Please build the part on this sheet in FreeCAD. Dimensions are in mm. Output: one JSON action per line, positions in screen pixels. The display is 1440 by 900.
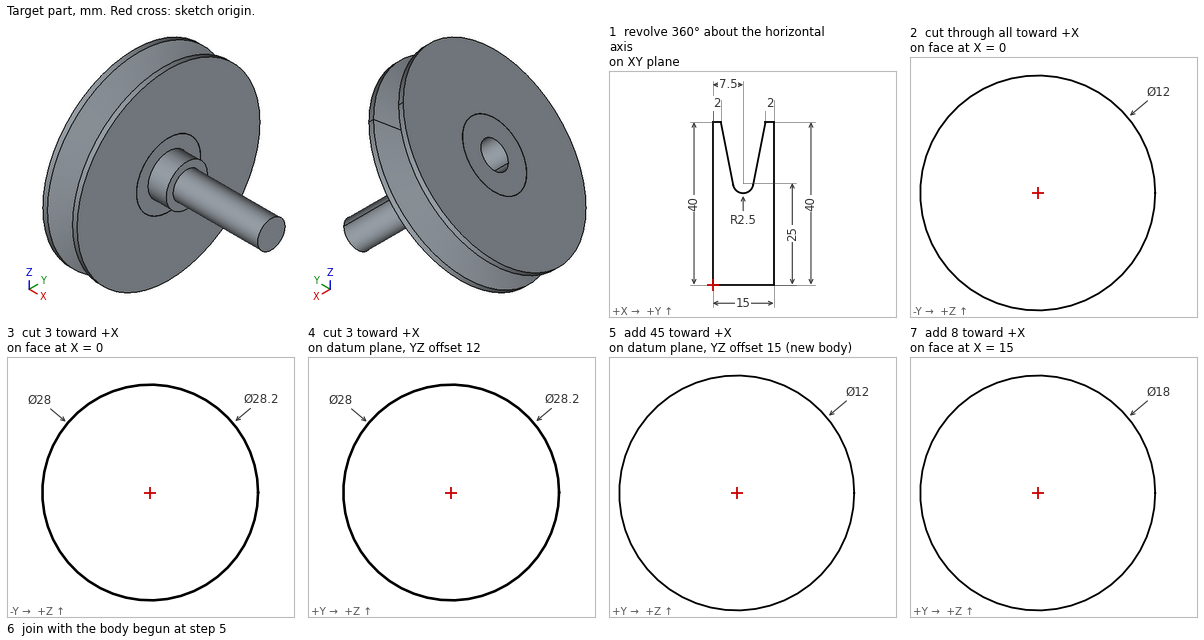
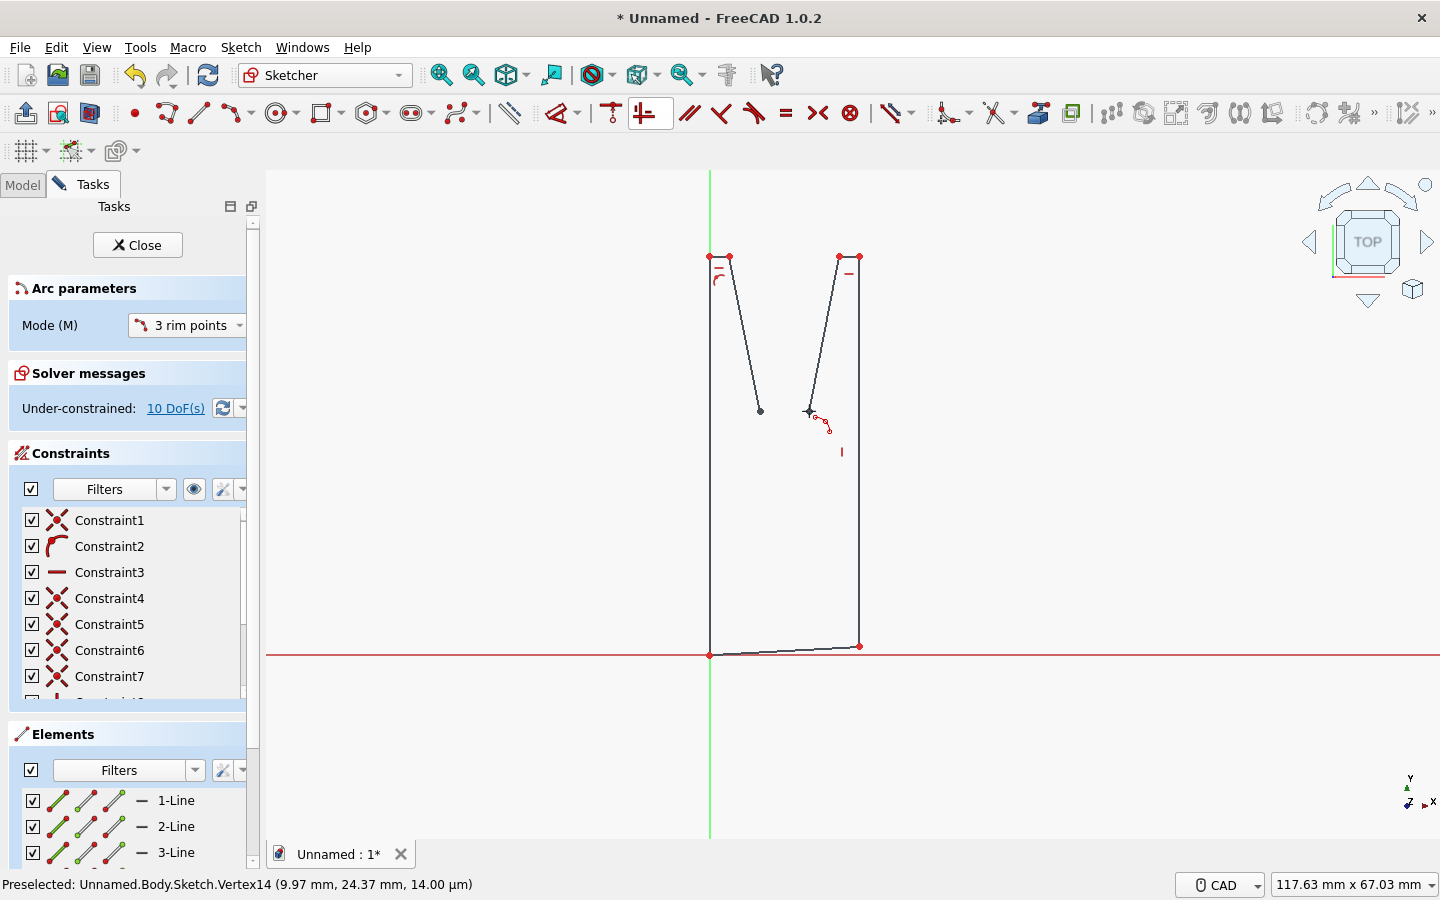
{"action": "left_click", "coordinate": [809, 412]}
{"action": "left_click", "coordinate": [760, 412]}
{"action": "left_click", "coordinate": [784, 431]}
{"action": "key", "text": "Escape"}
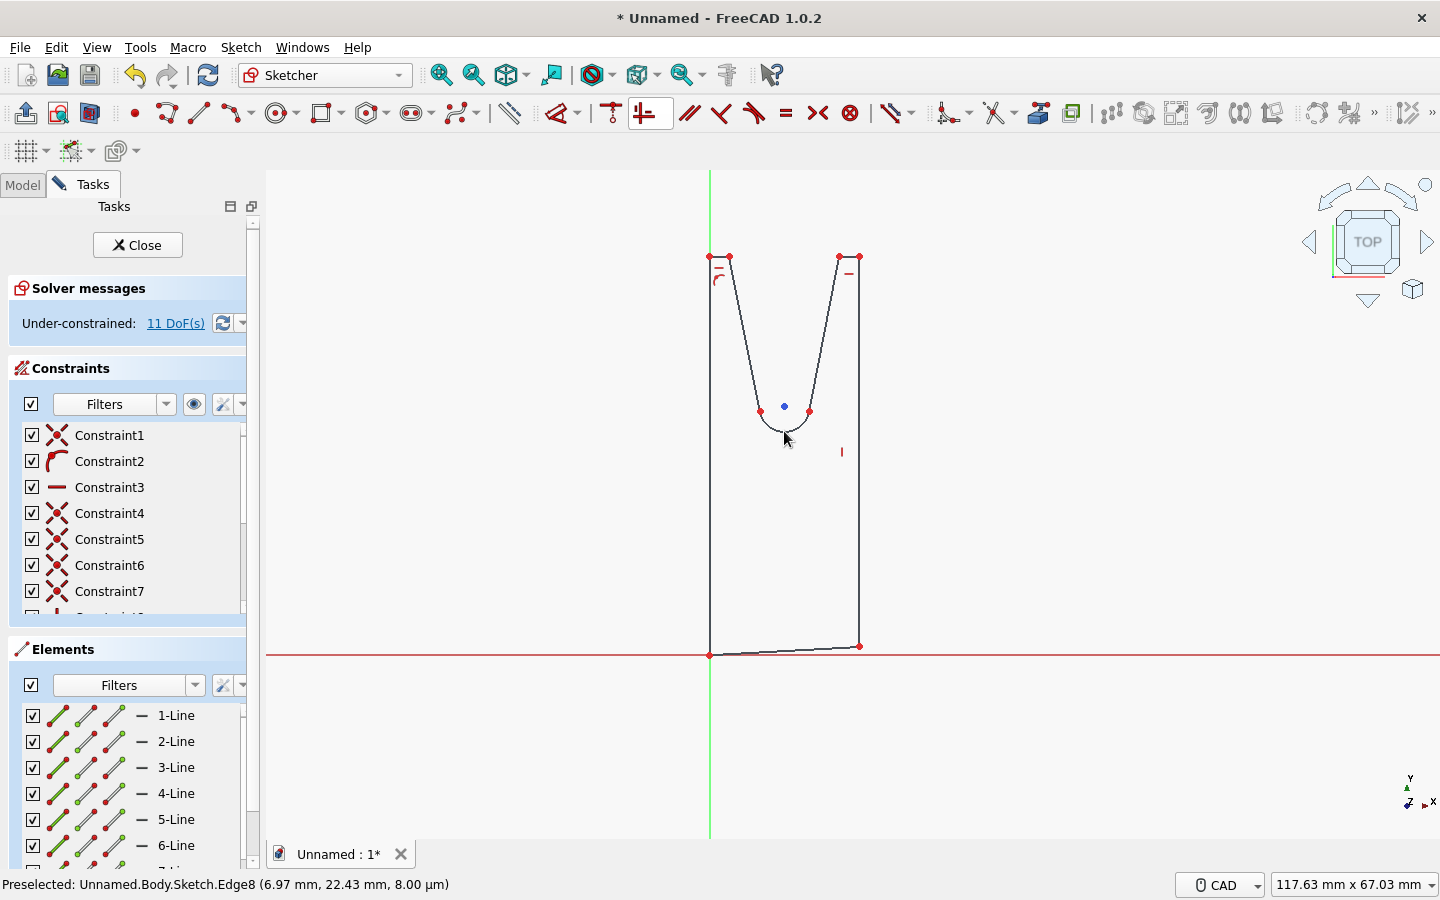
{"action": "left_click", "coordinate": [751, 365]}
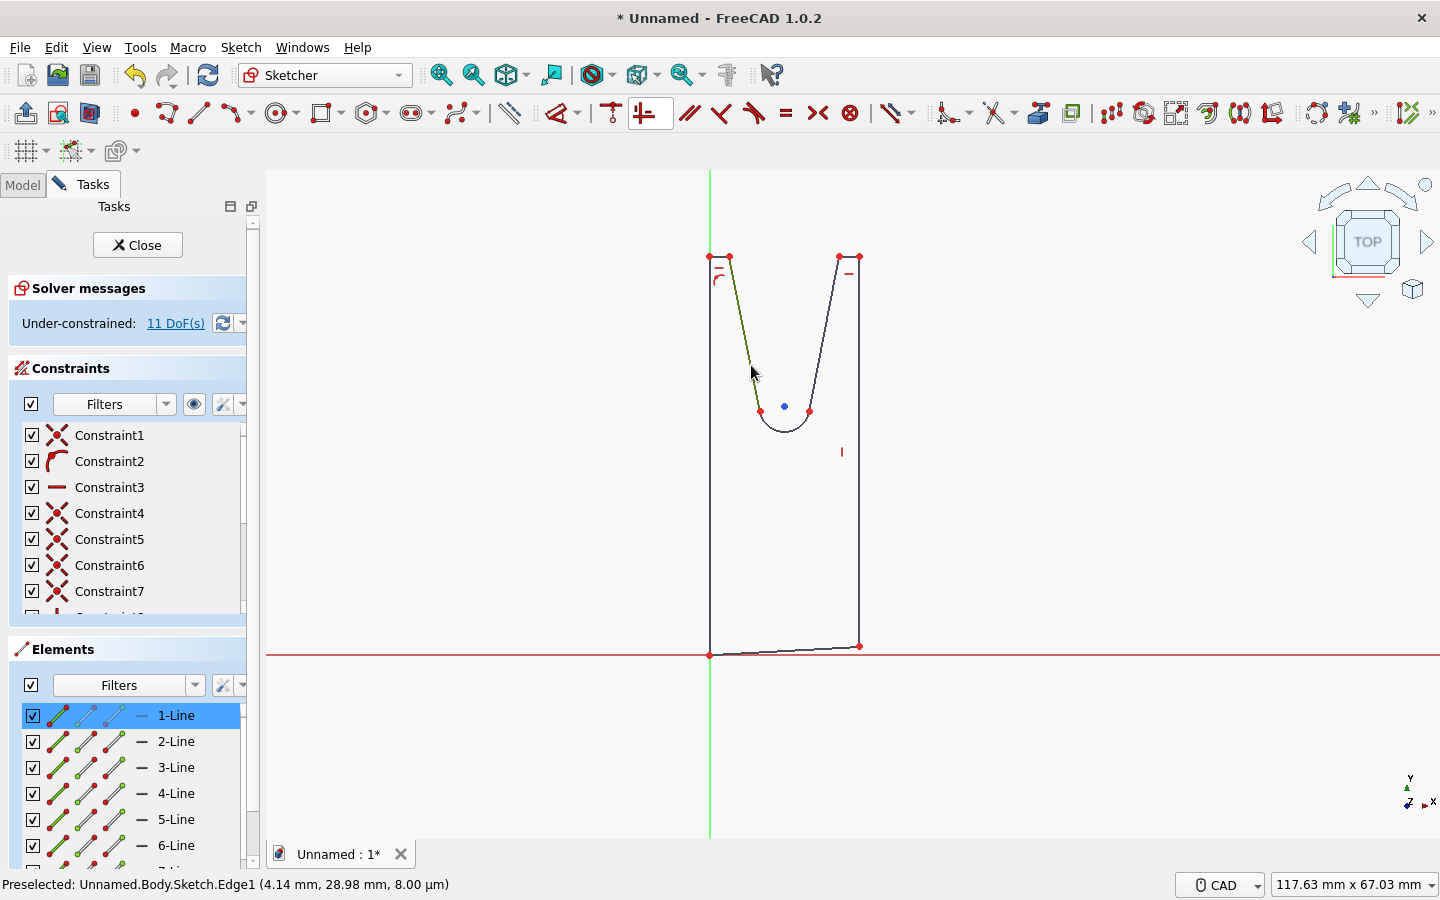
{"action": "left_click", "coordinate": [771, 428]}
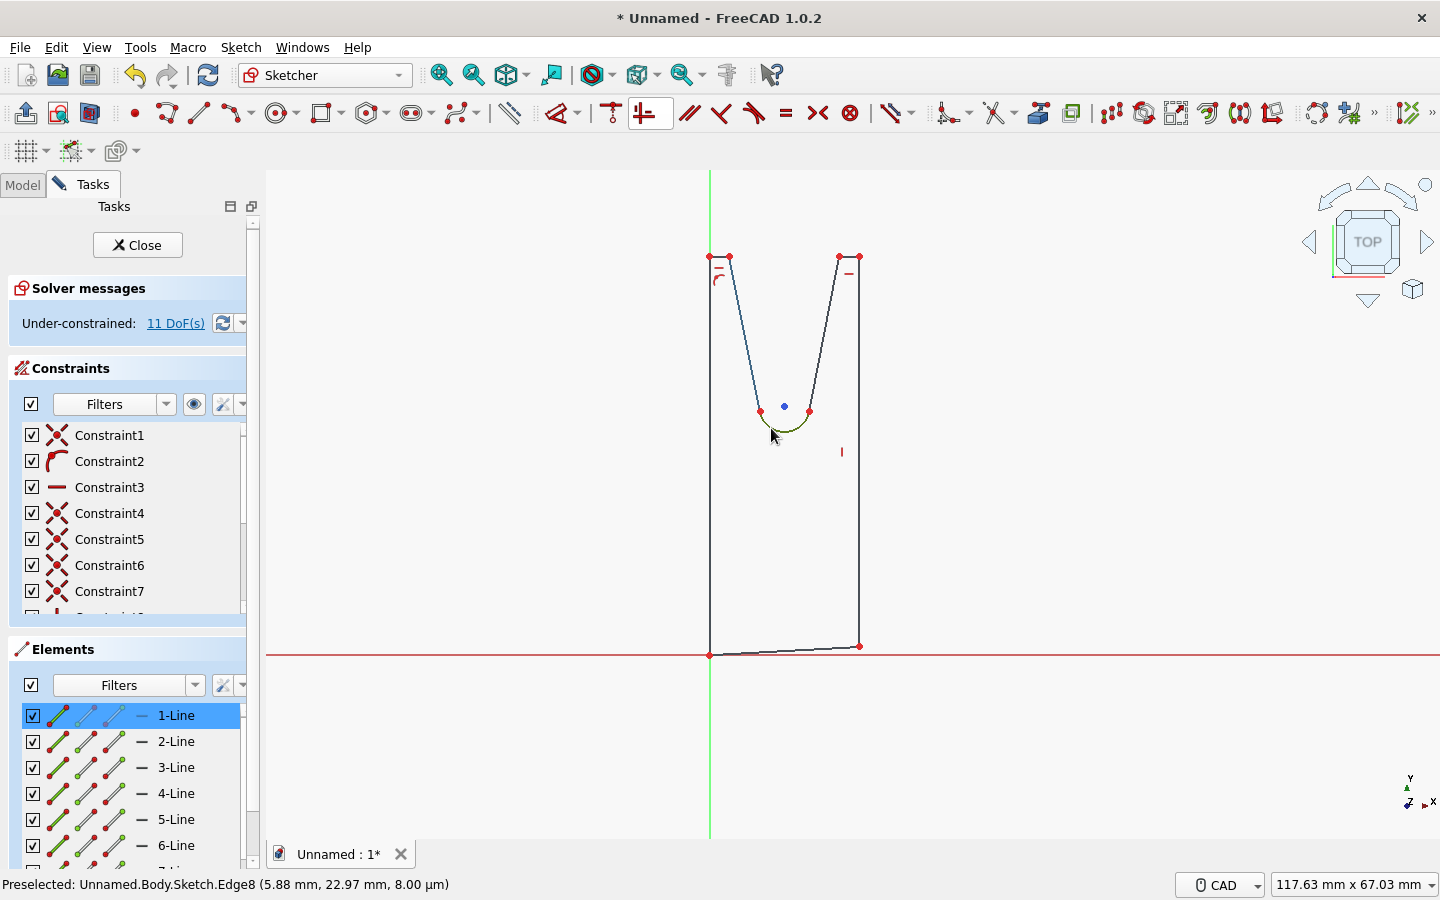
{"action": "key", "text": "t"}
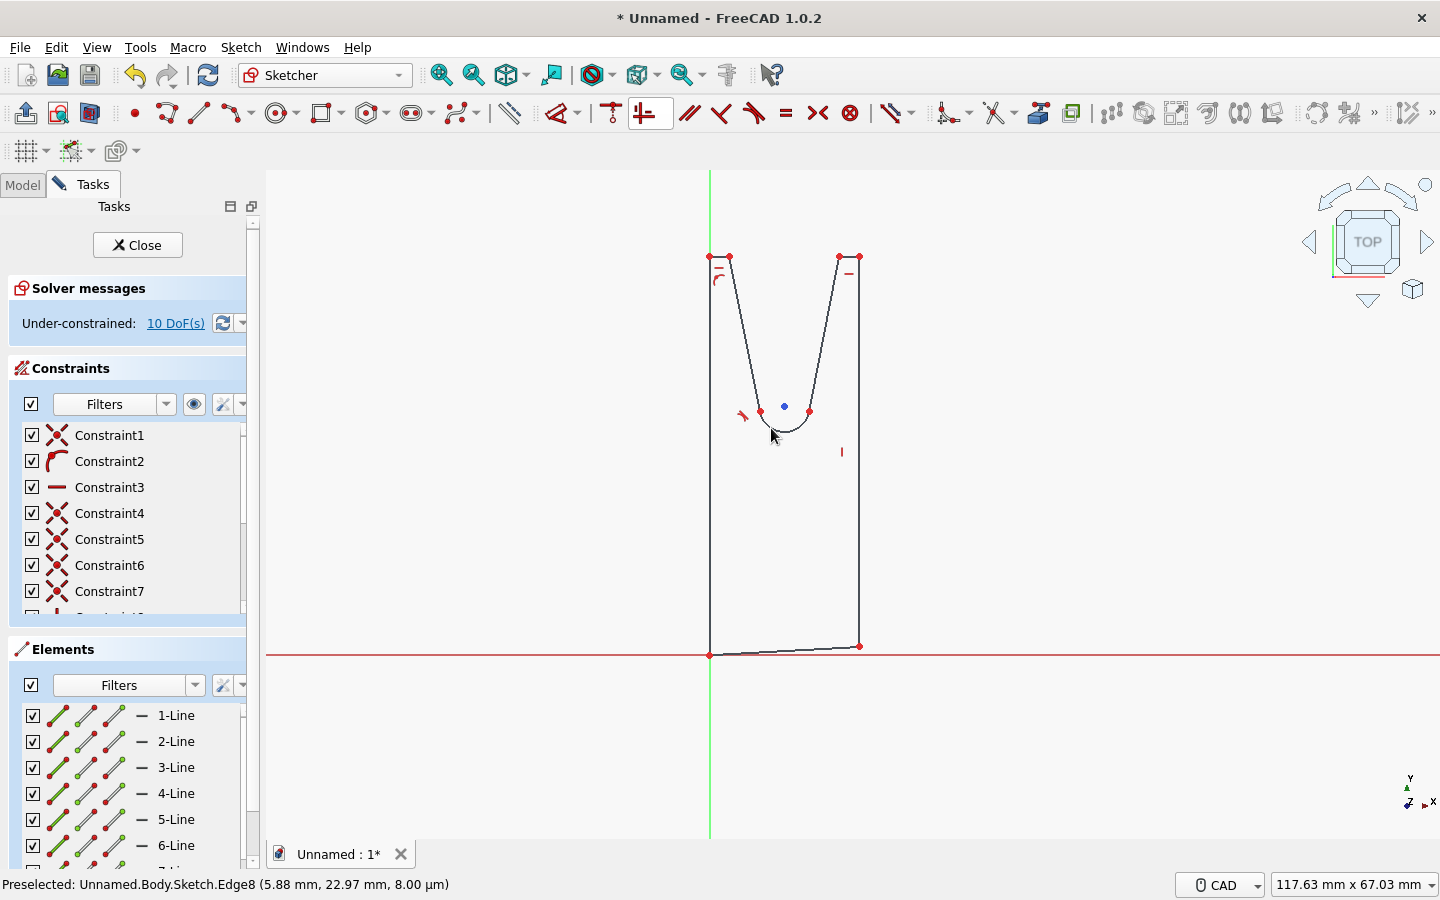
{"action": "left_click", "coordinate": [830, 303]}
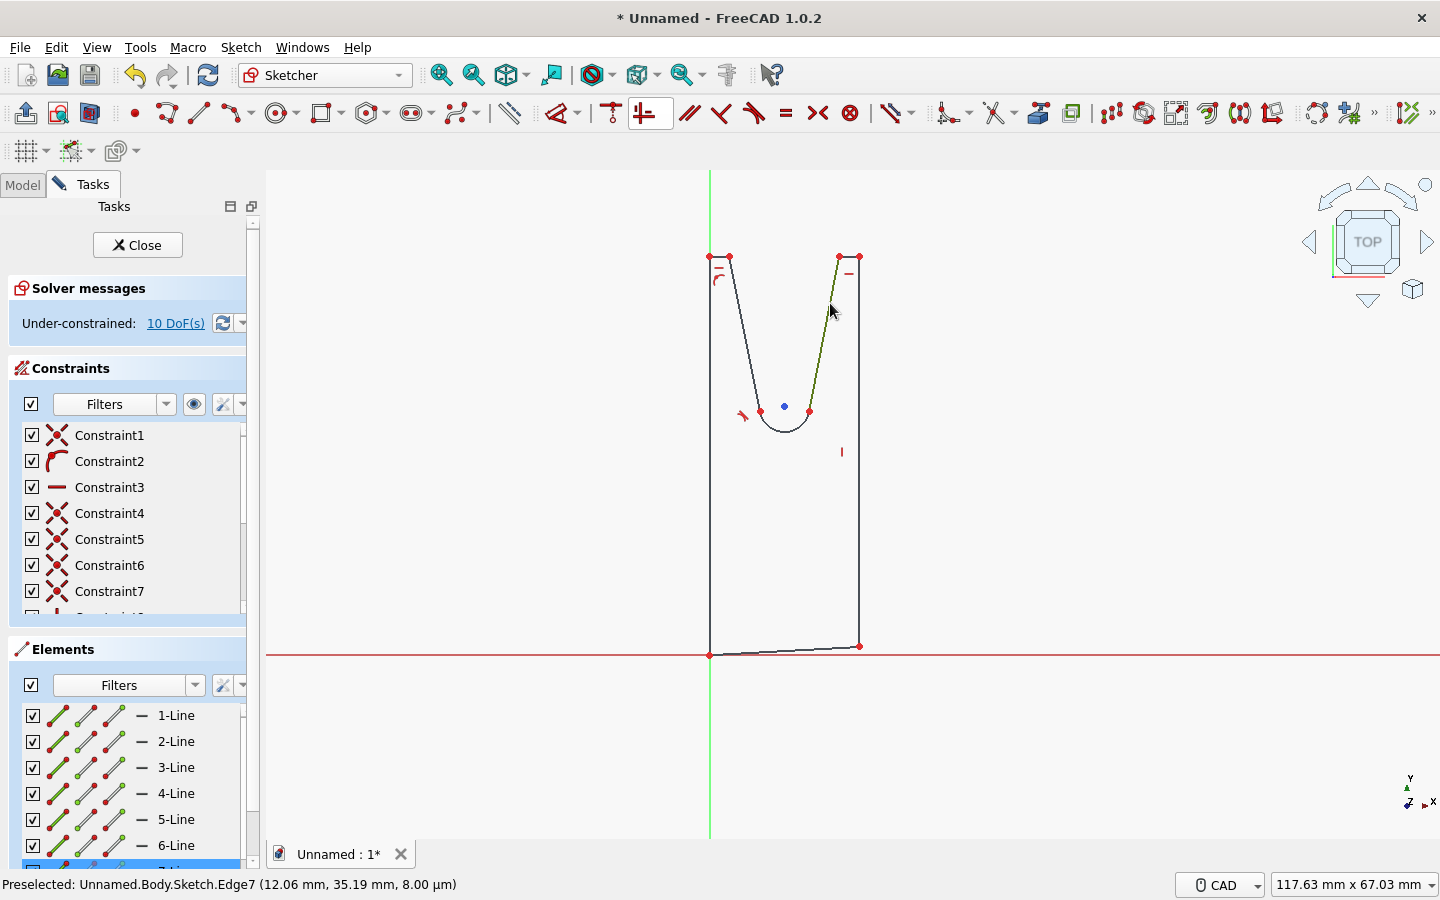
{"action": "left_click", "coordinate": [771, 428]}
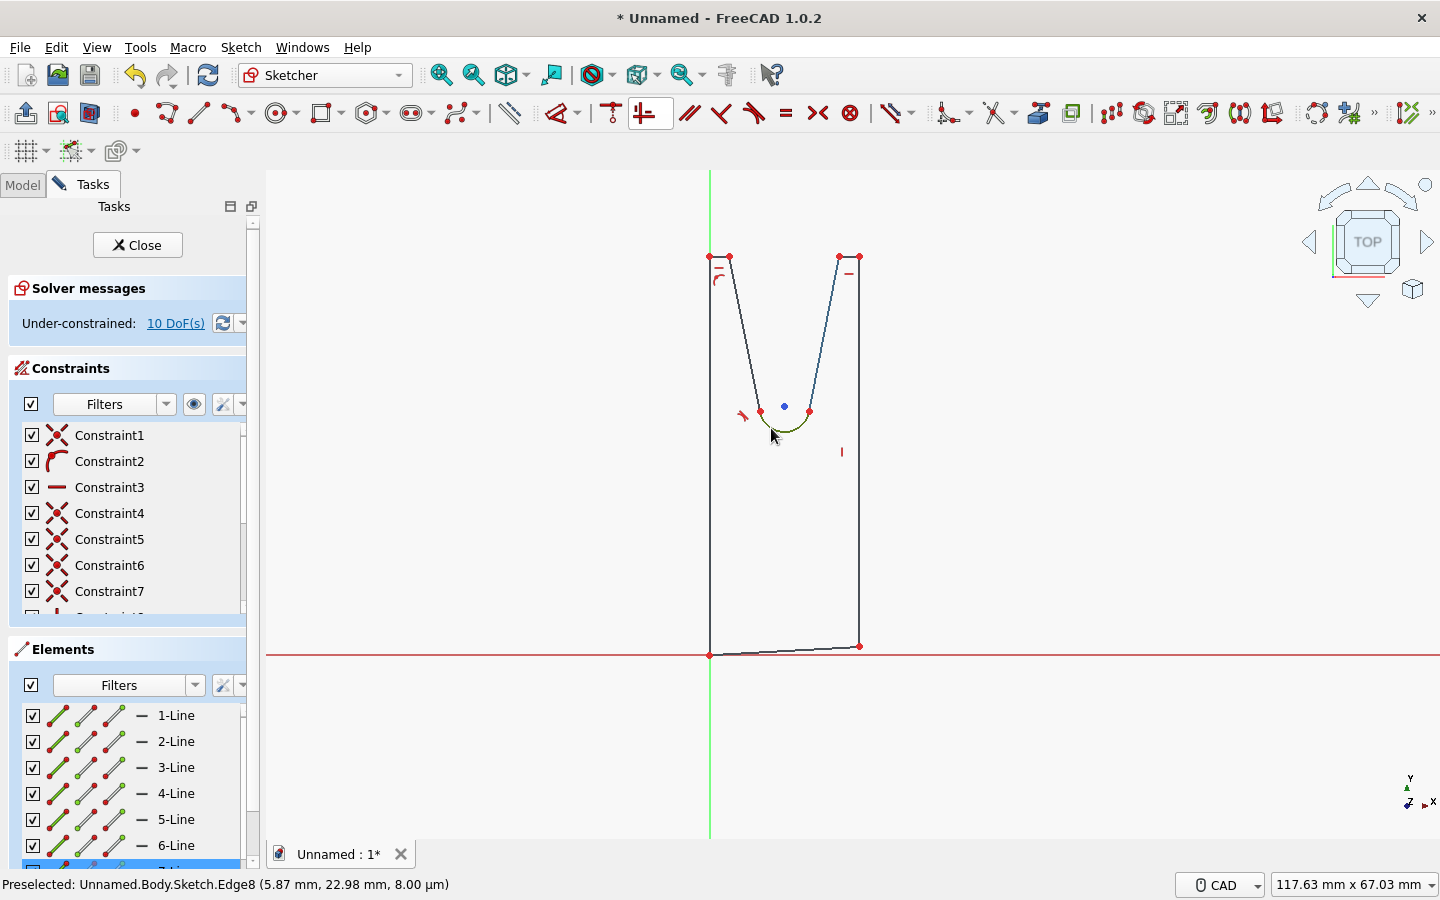
{"action": "left_click", "coordinate": [754, 114]}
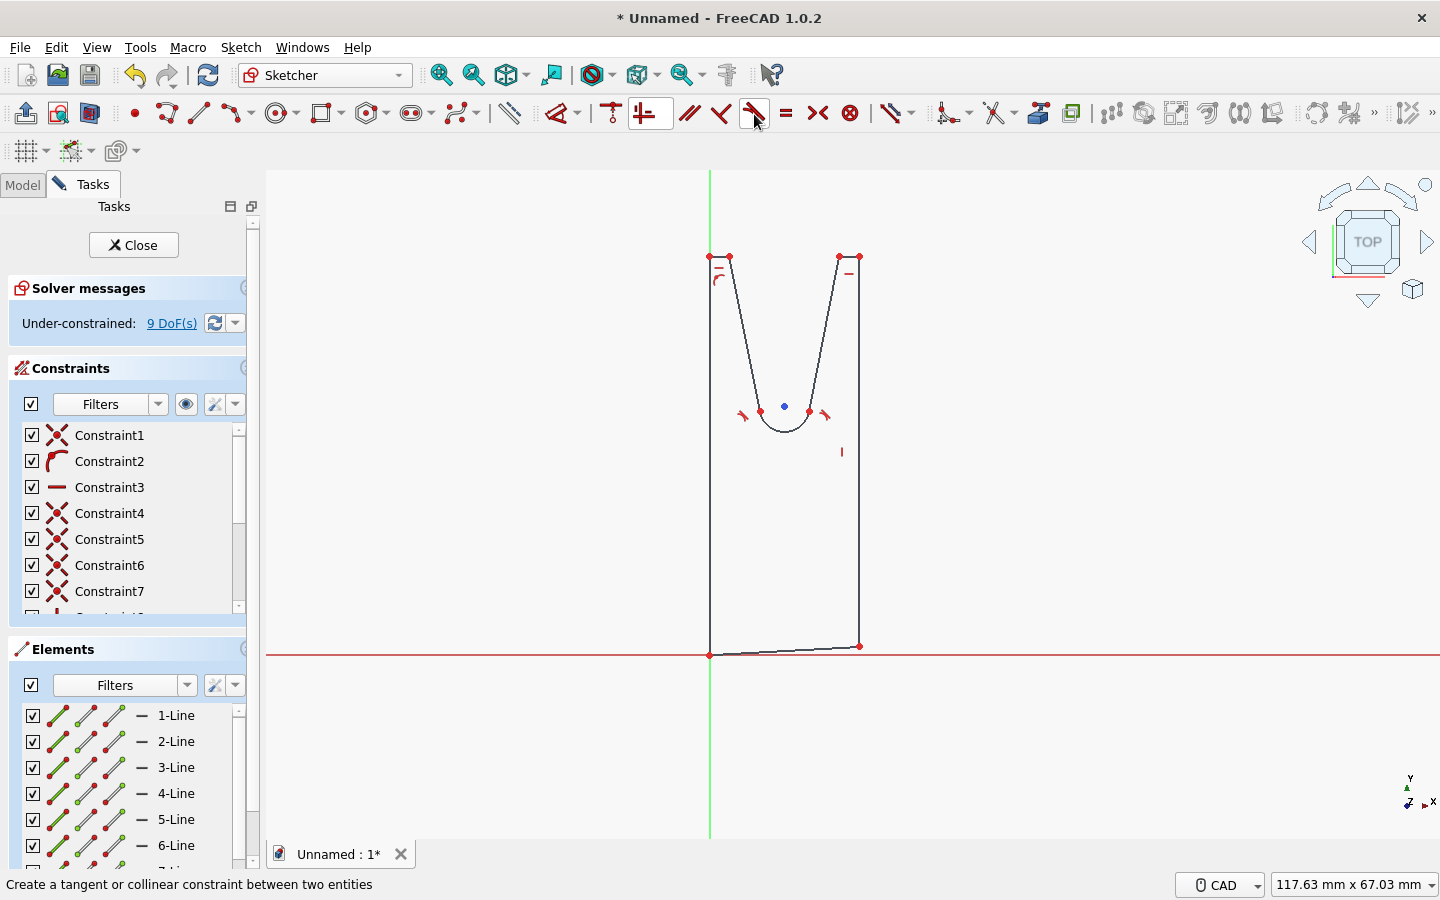
{"action": "left_click", "coordinate": [754, 653]}